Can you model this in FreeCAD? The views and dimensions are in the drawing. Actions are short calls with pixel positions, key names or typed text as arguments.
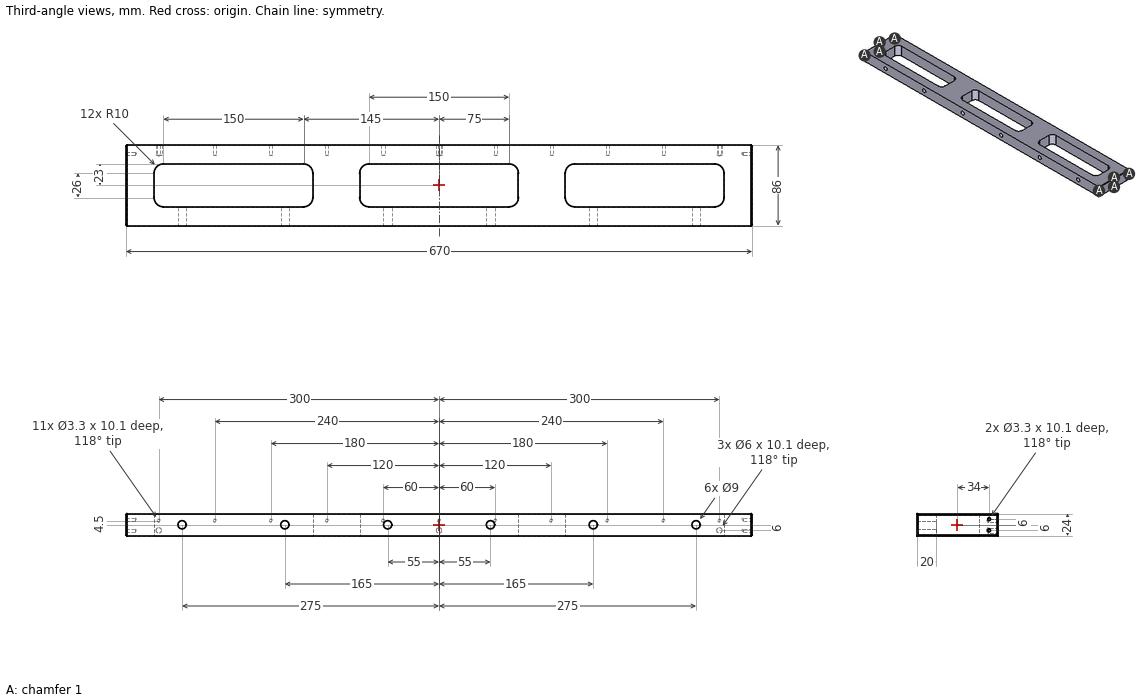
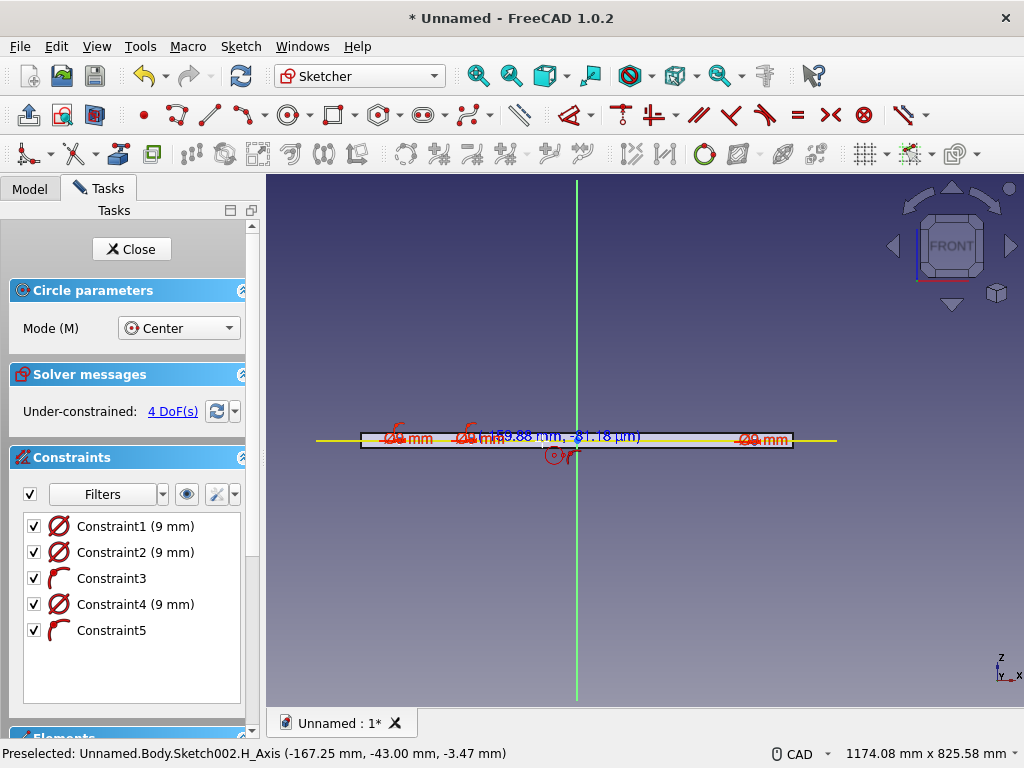
click(542, 441)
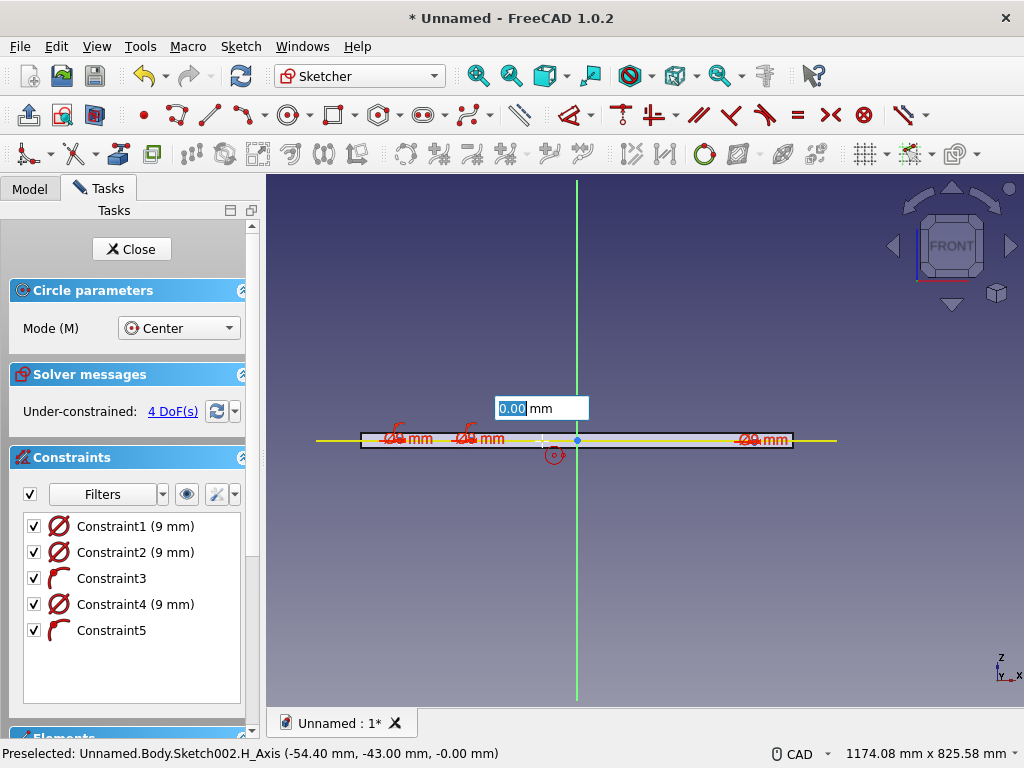
scroll(541, 443, up, 9)
move(537, 443)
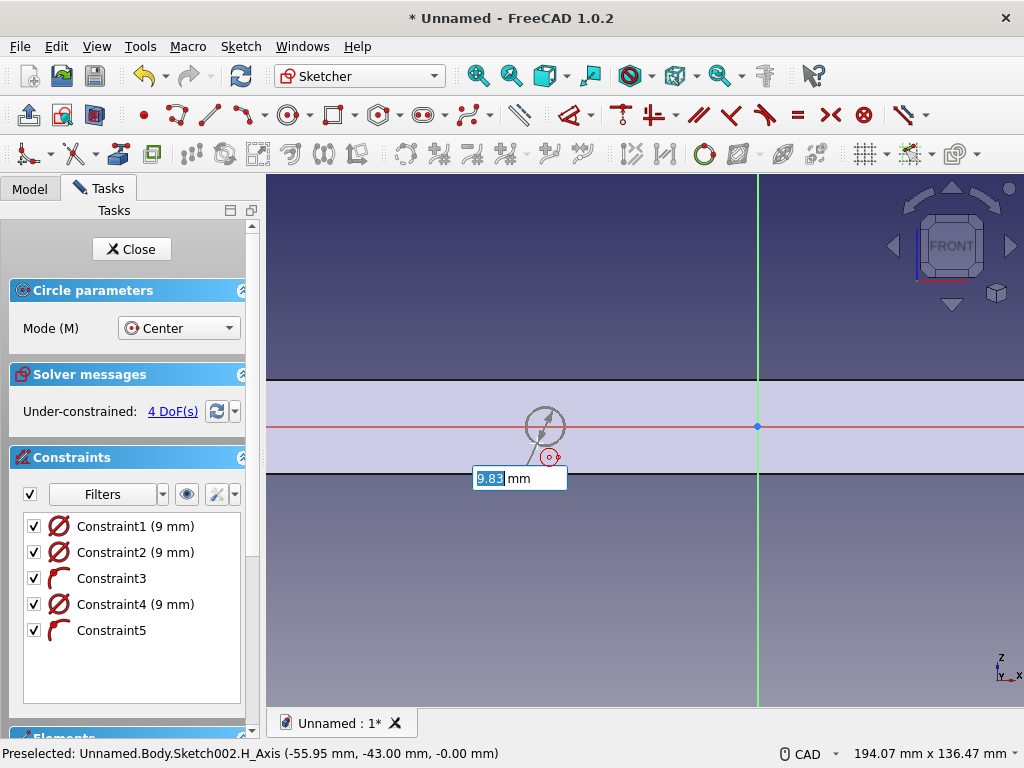
text(9)
key(Return)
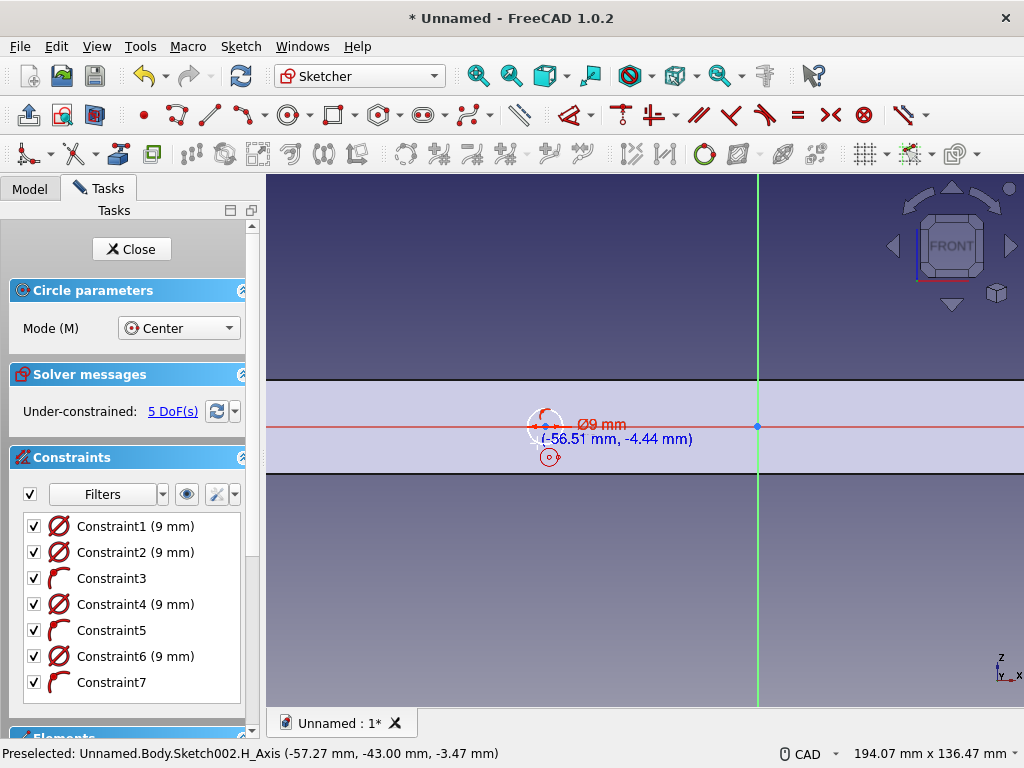
scroll(541, 443, down, 9)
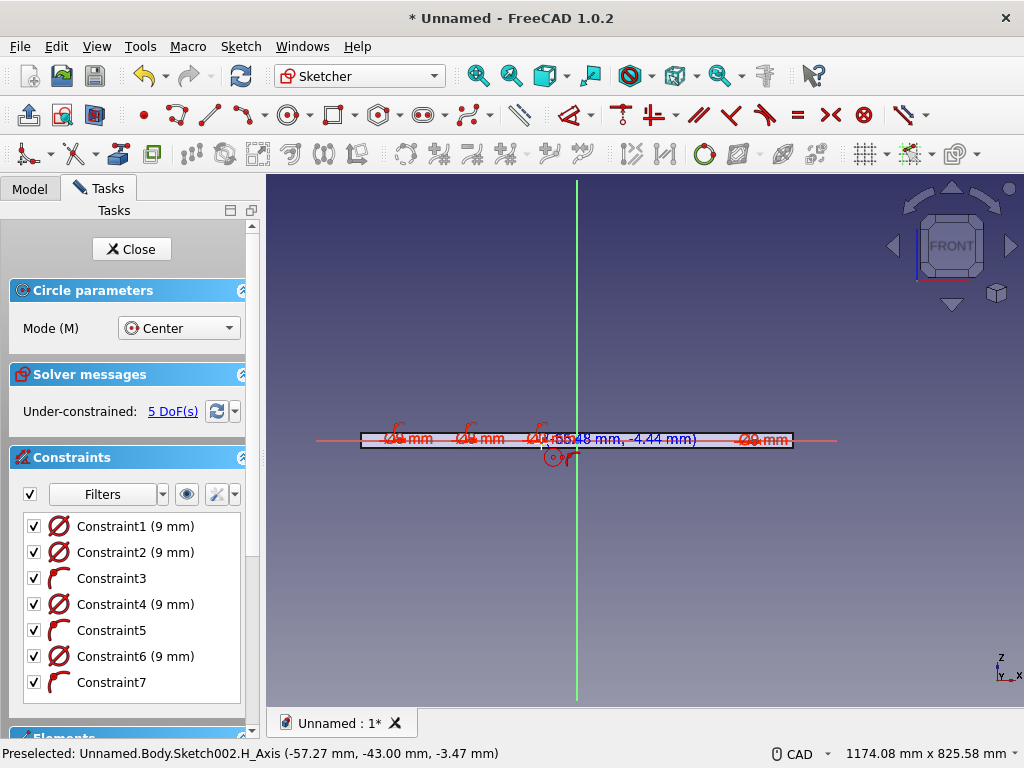
scroll(613, 441, up, 11)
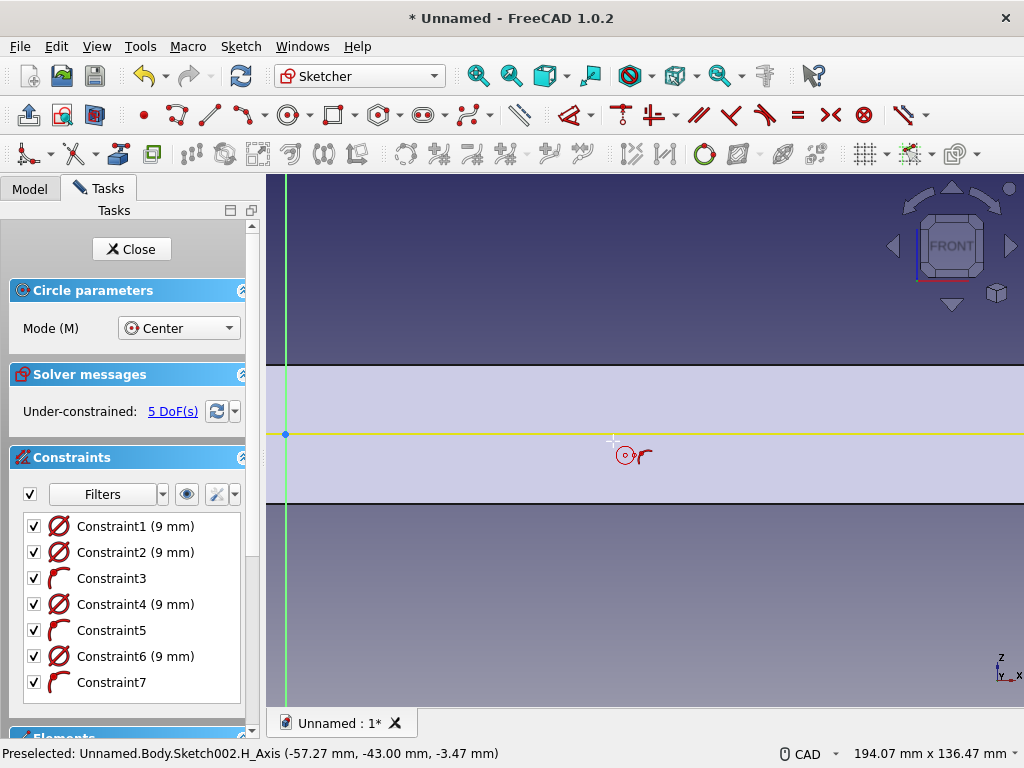
scroll(613, 441, down, 11)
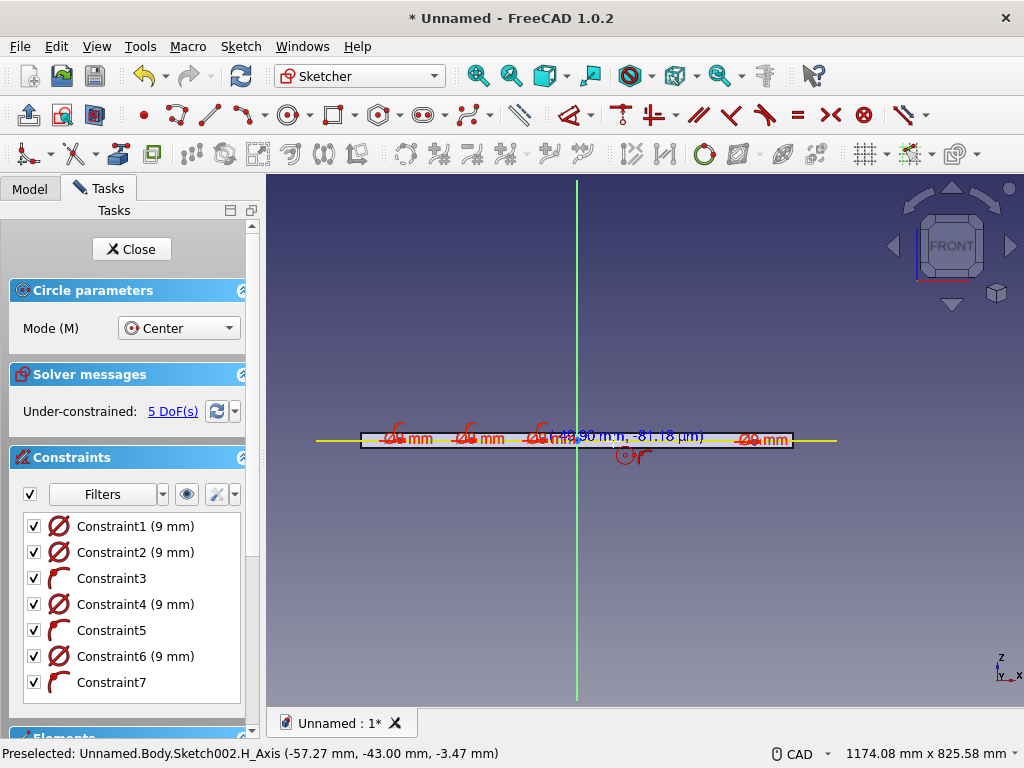
click(613, 441)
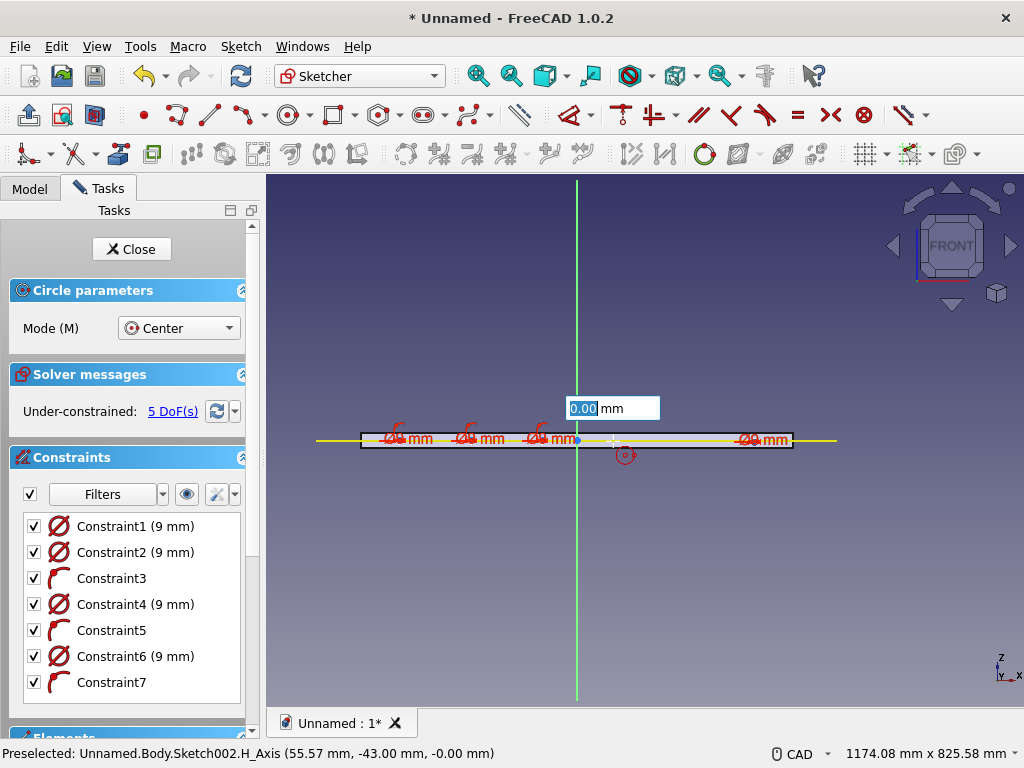
scroll(612, 443, up, 9)
move(608, 443)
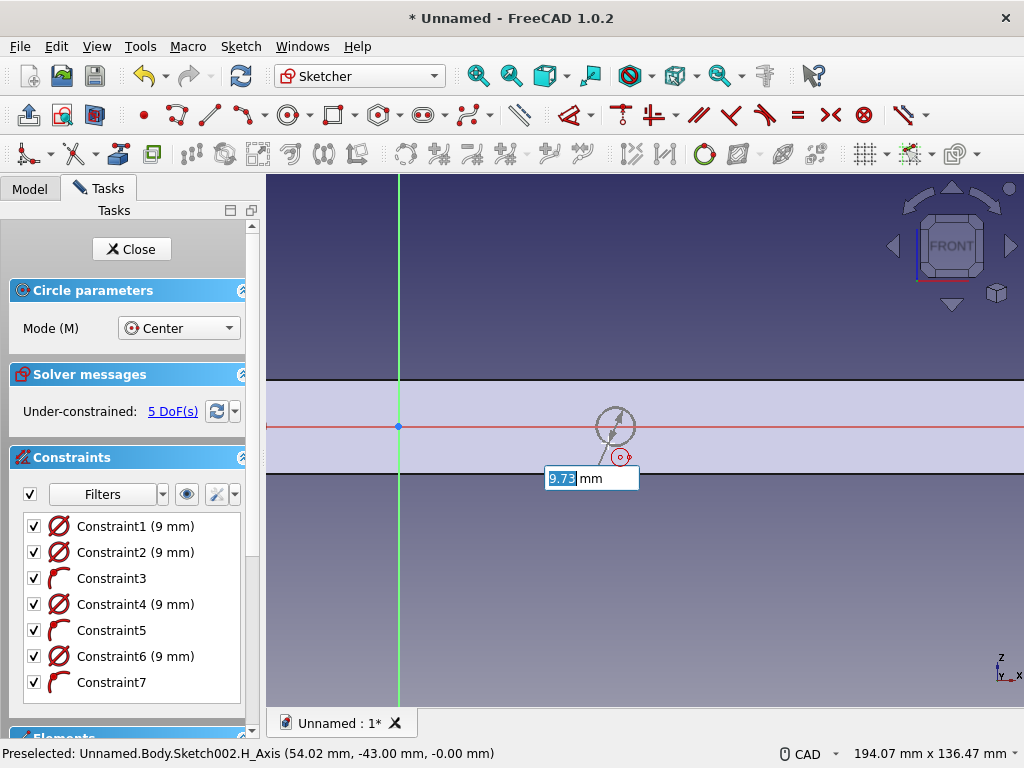
text(9)
key(Return)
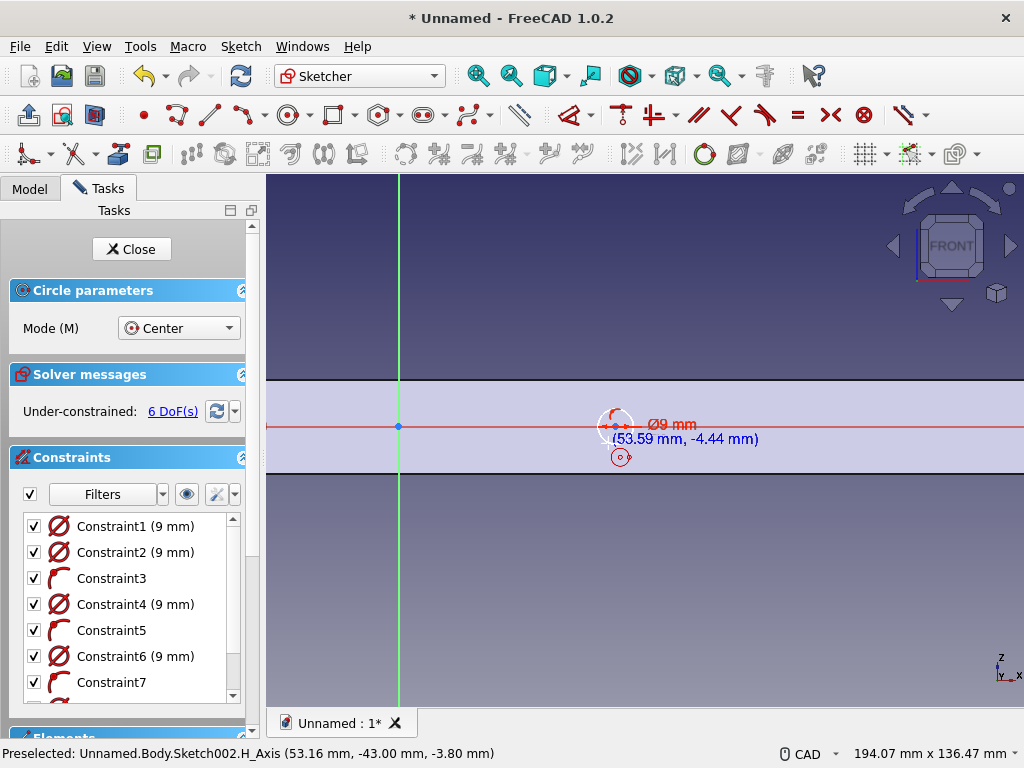
scroll(612, 443, down, 9)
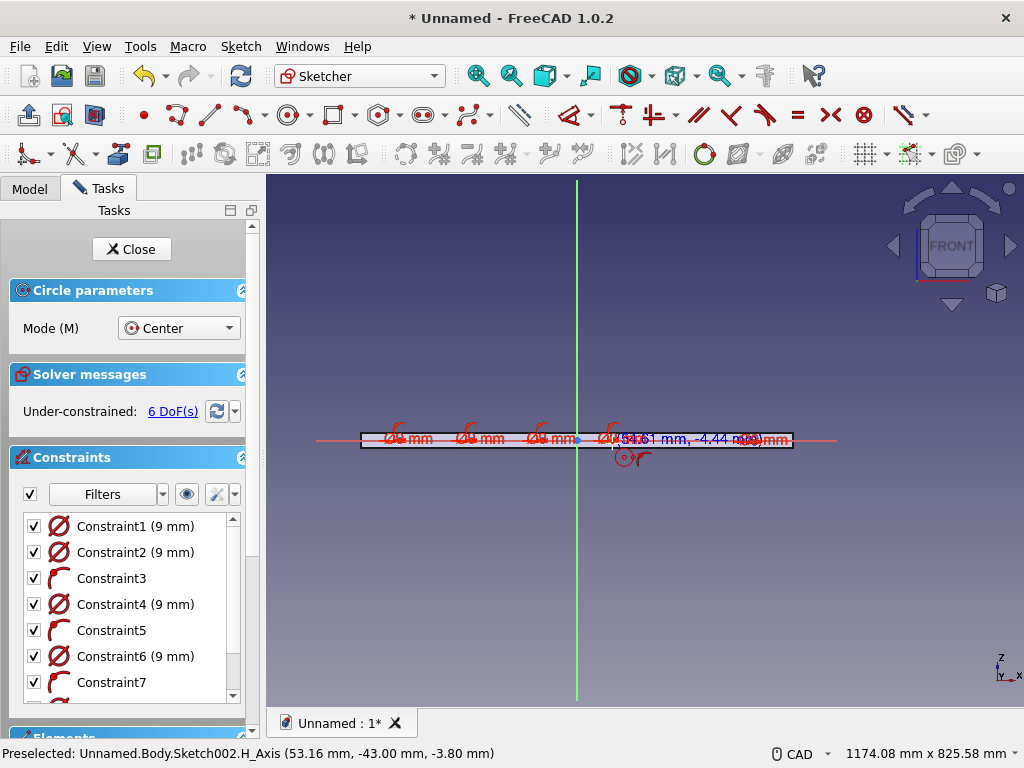
scroll(684, 441, up, 11)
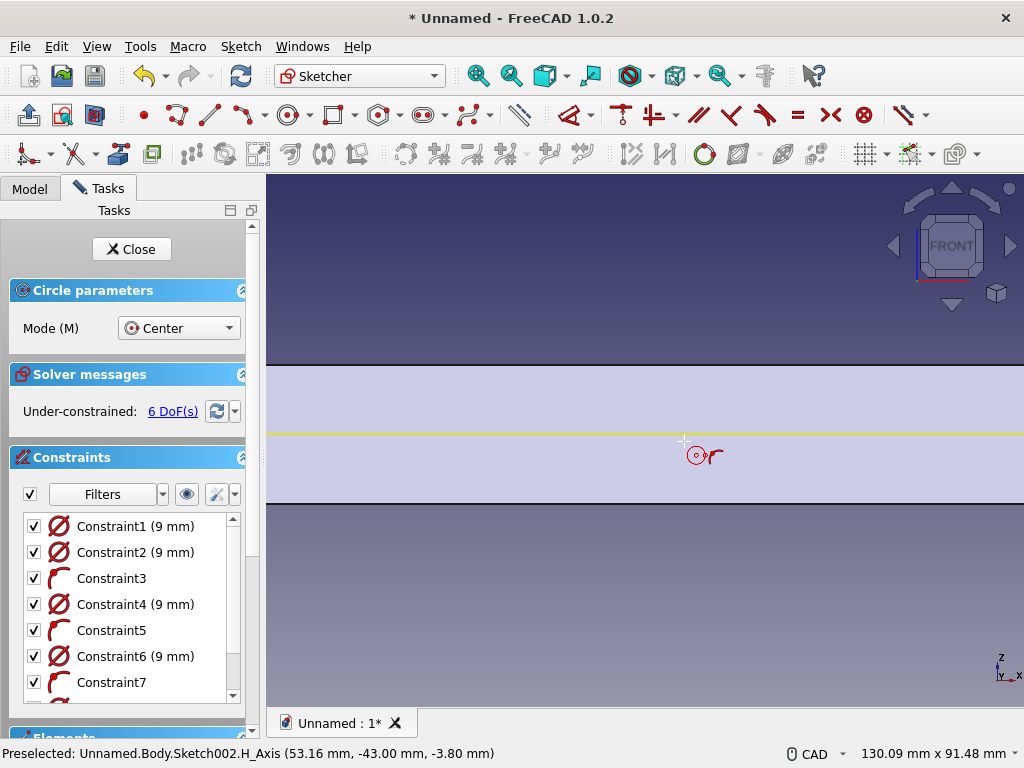
scroll(684, 441, down, 11)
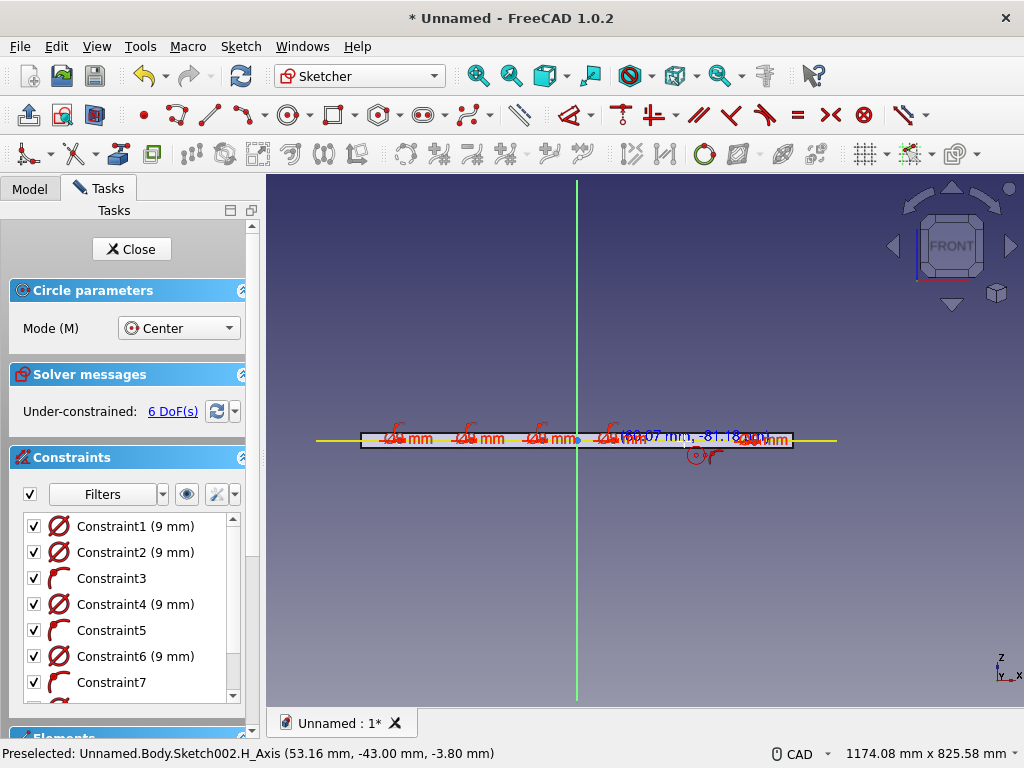
click(684, 441)